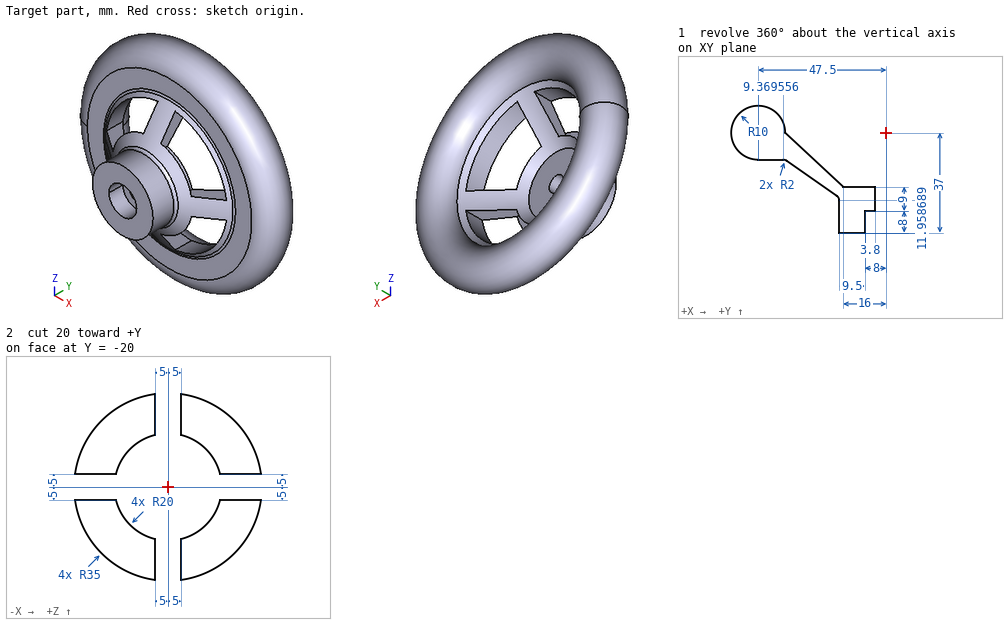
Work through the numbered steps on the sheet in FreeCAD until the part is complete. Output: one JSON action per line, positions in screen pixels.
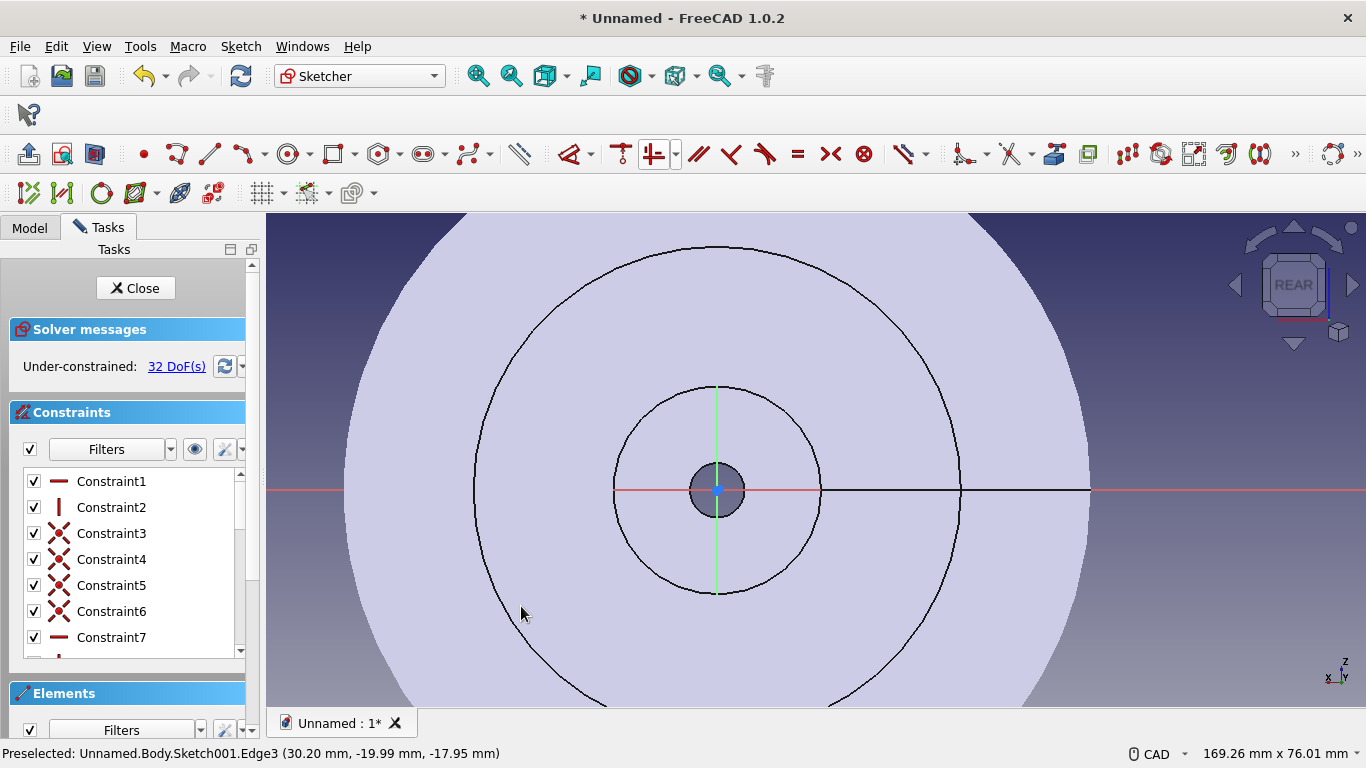
{"action": "left_click", "coordinate": [608, 562]}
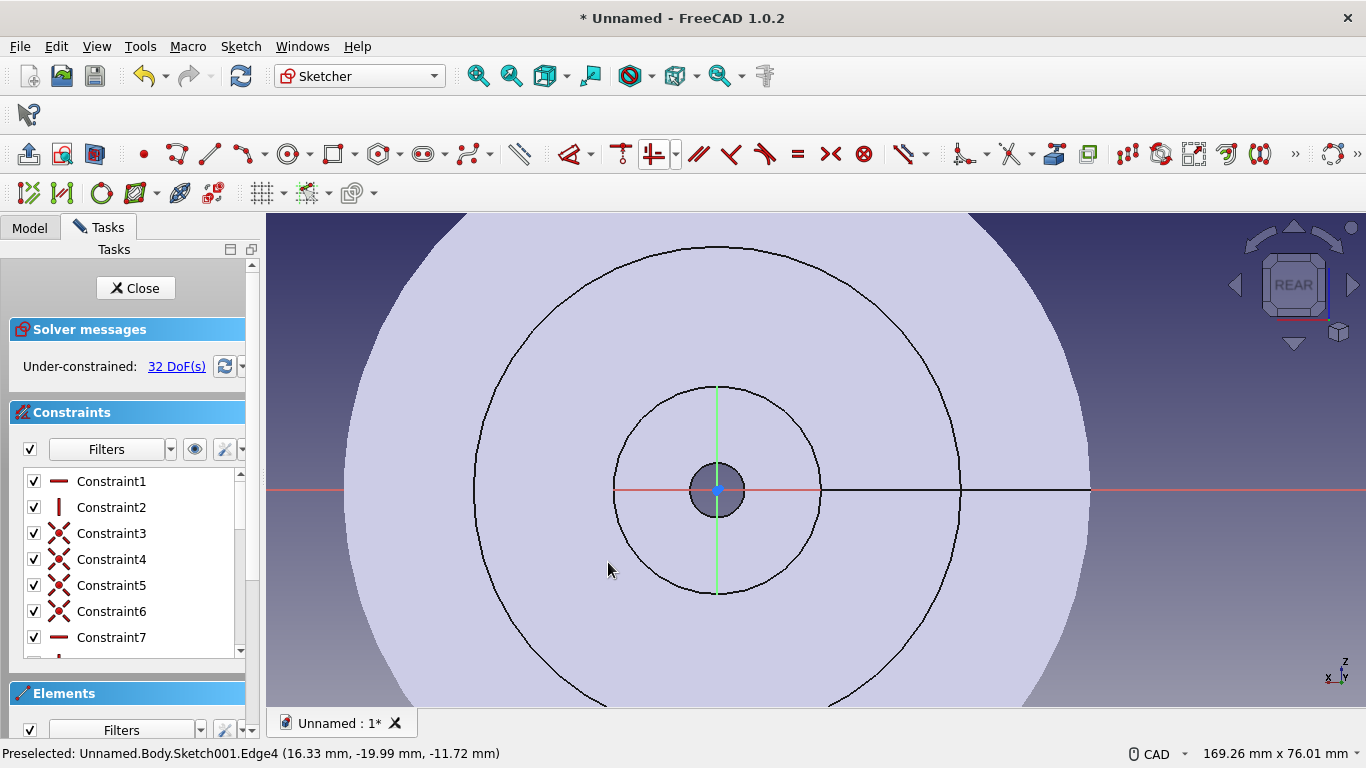
{"action": "key", "text": "c"}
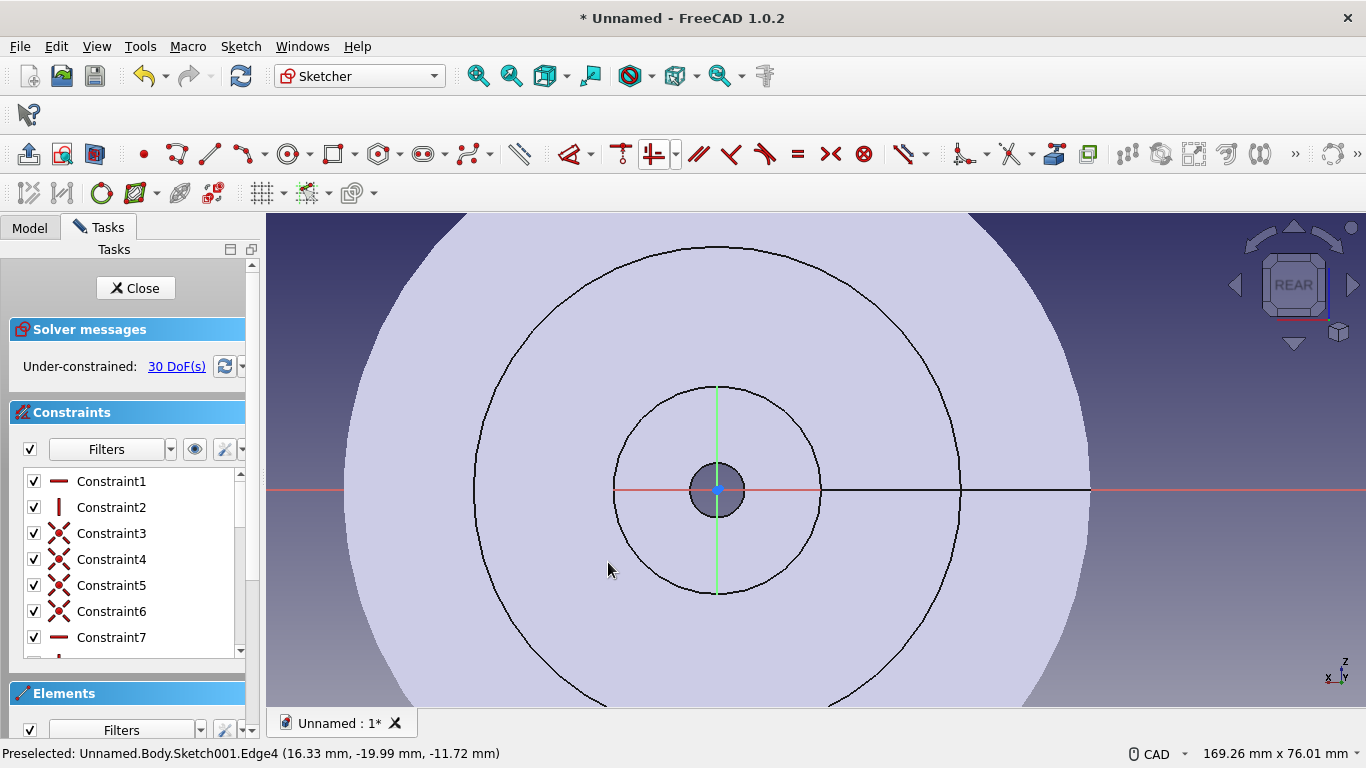
{"action": "left_click", "coordinate": [521, 606]}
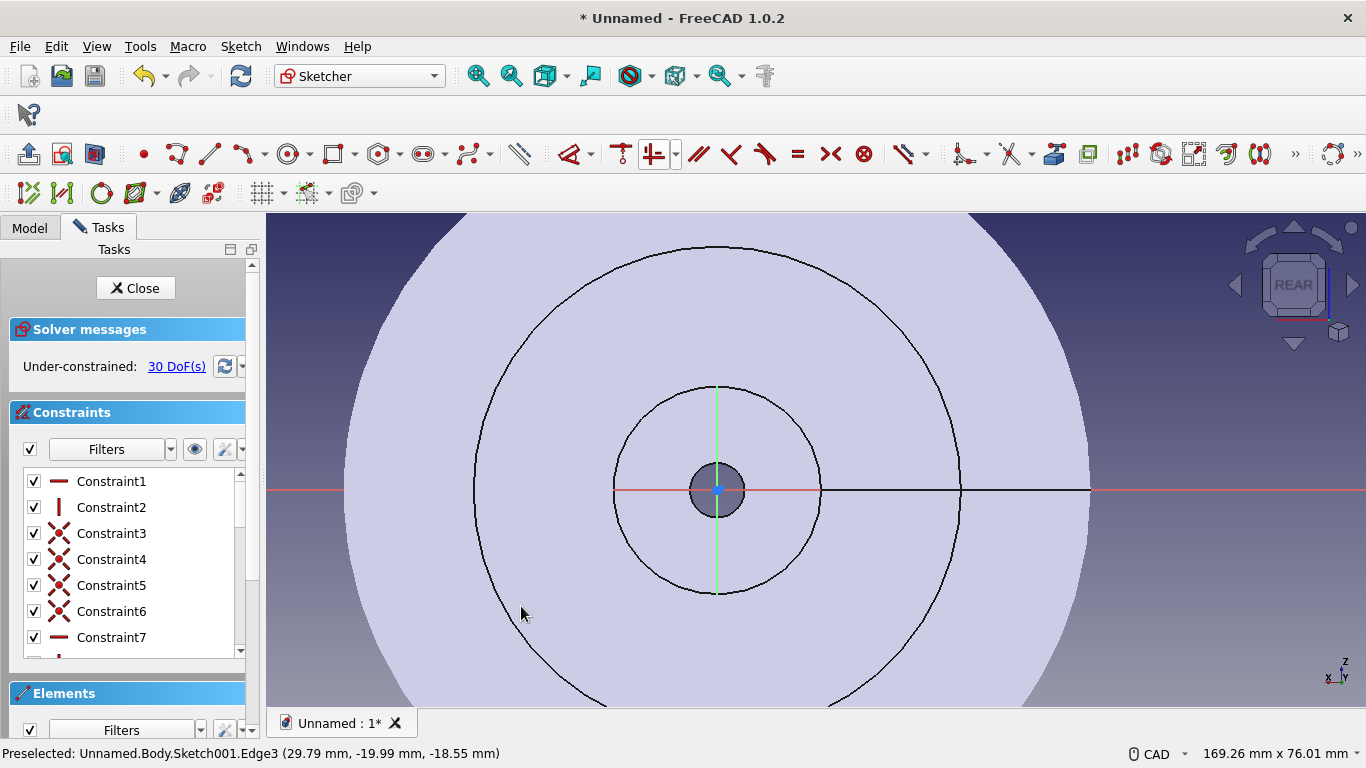
{"action": "left_click", "coordinate": [647, 382]}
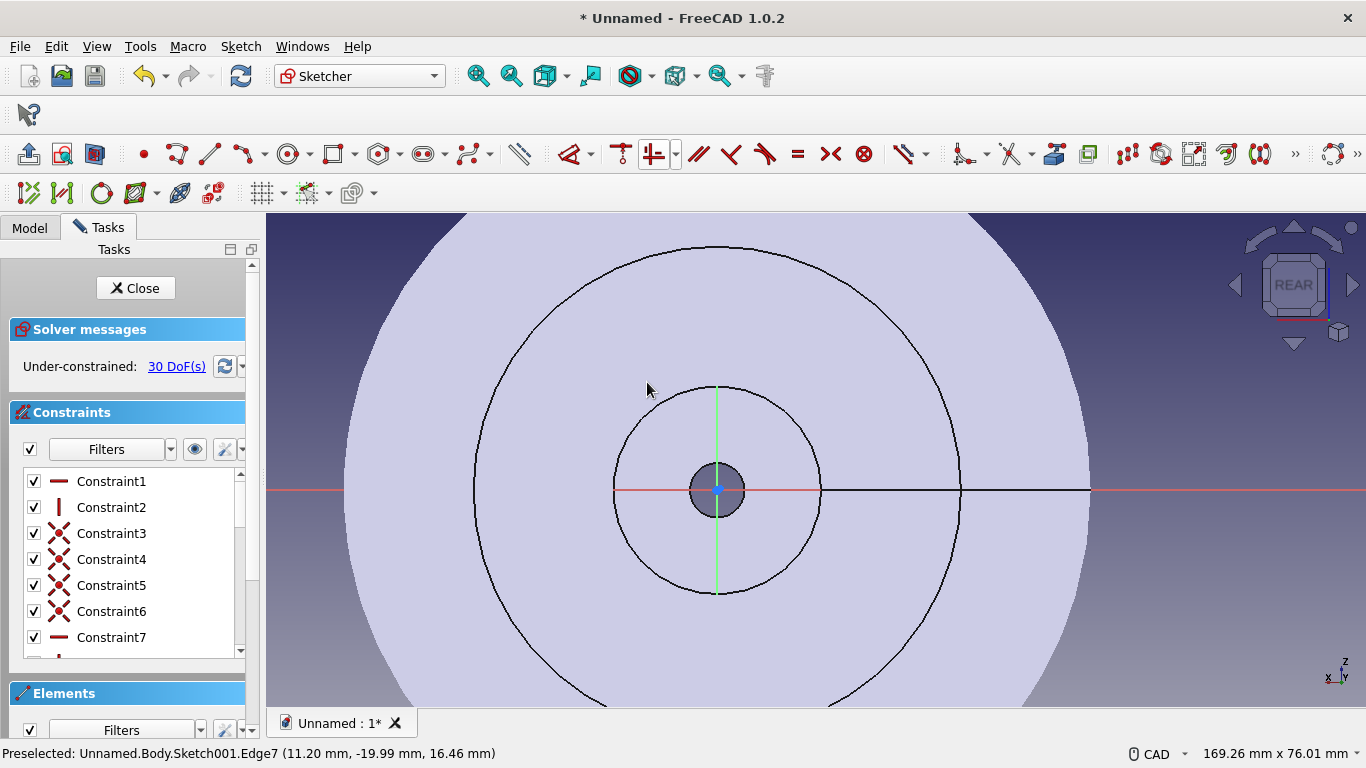
{"action": "key", "text": "c"}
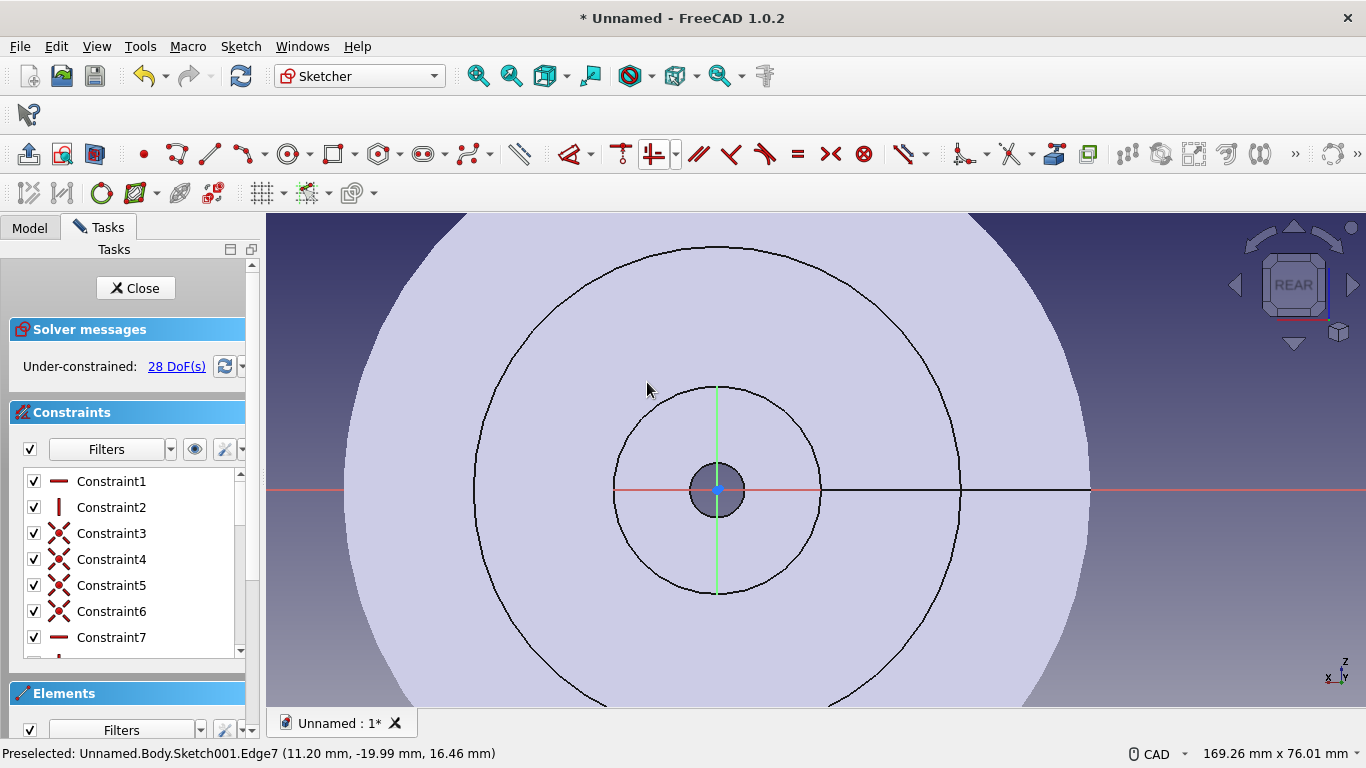
{"action": "left_click", "coordinate": [521, 606]}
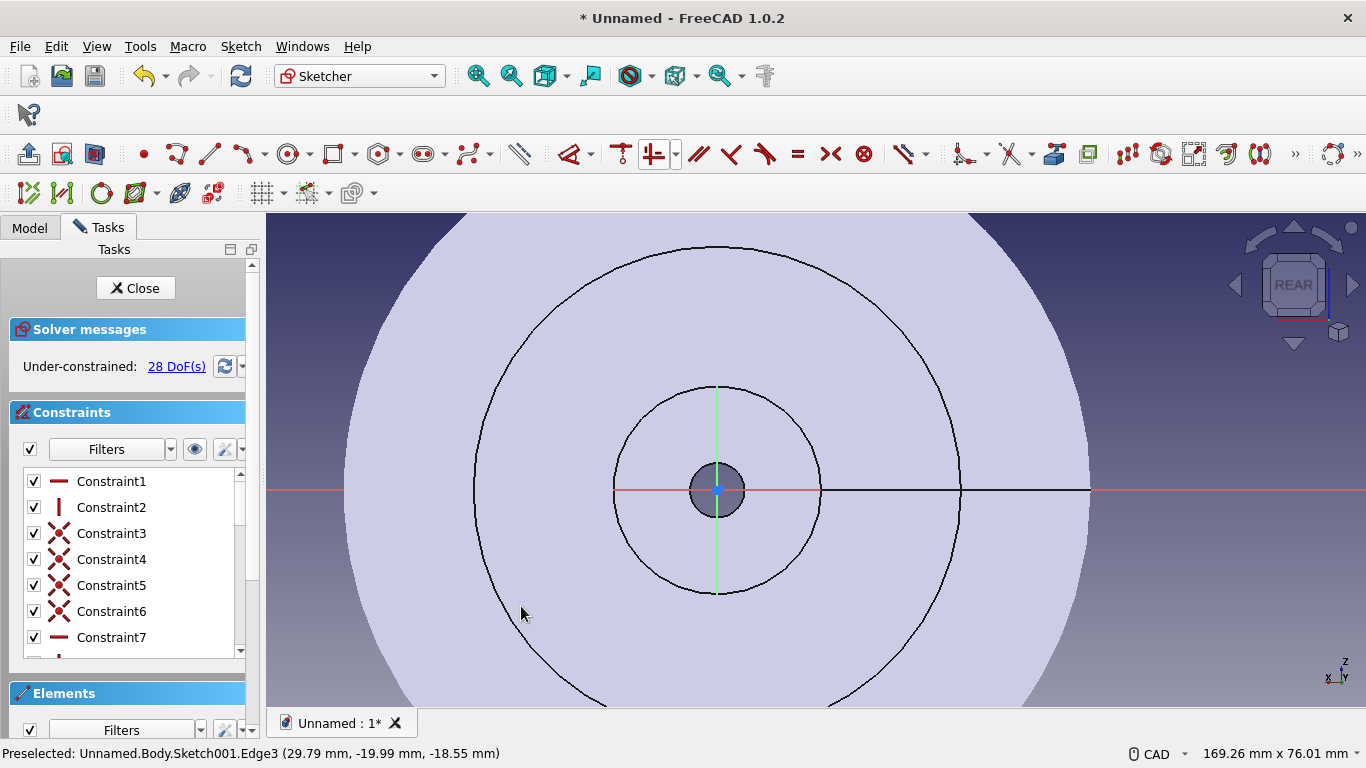
{"action": "left_click", "coordinate": [602, 295]}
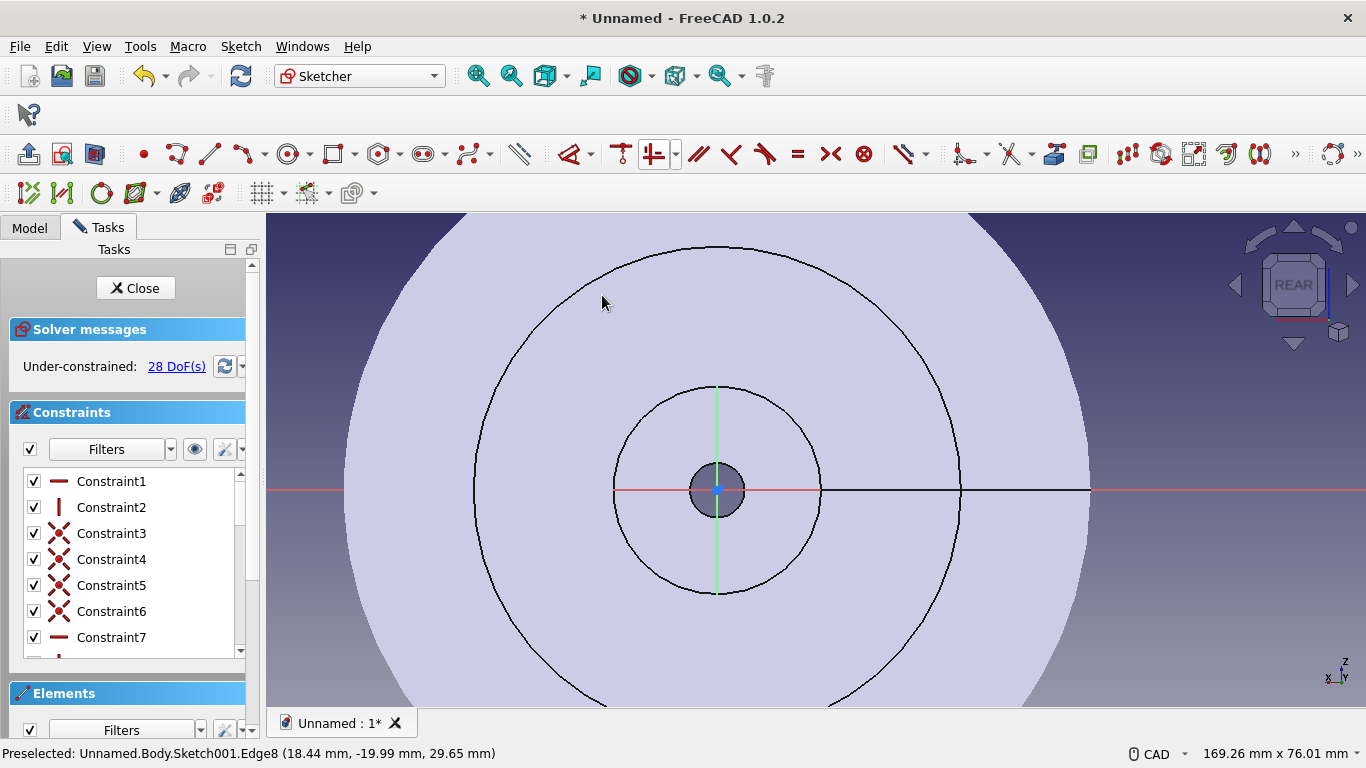
{"action": "key", "text": "c"}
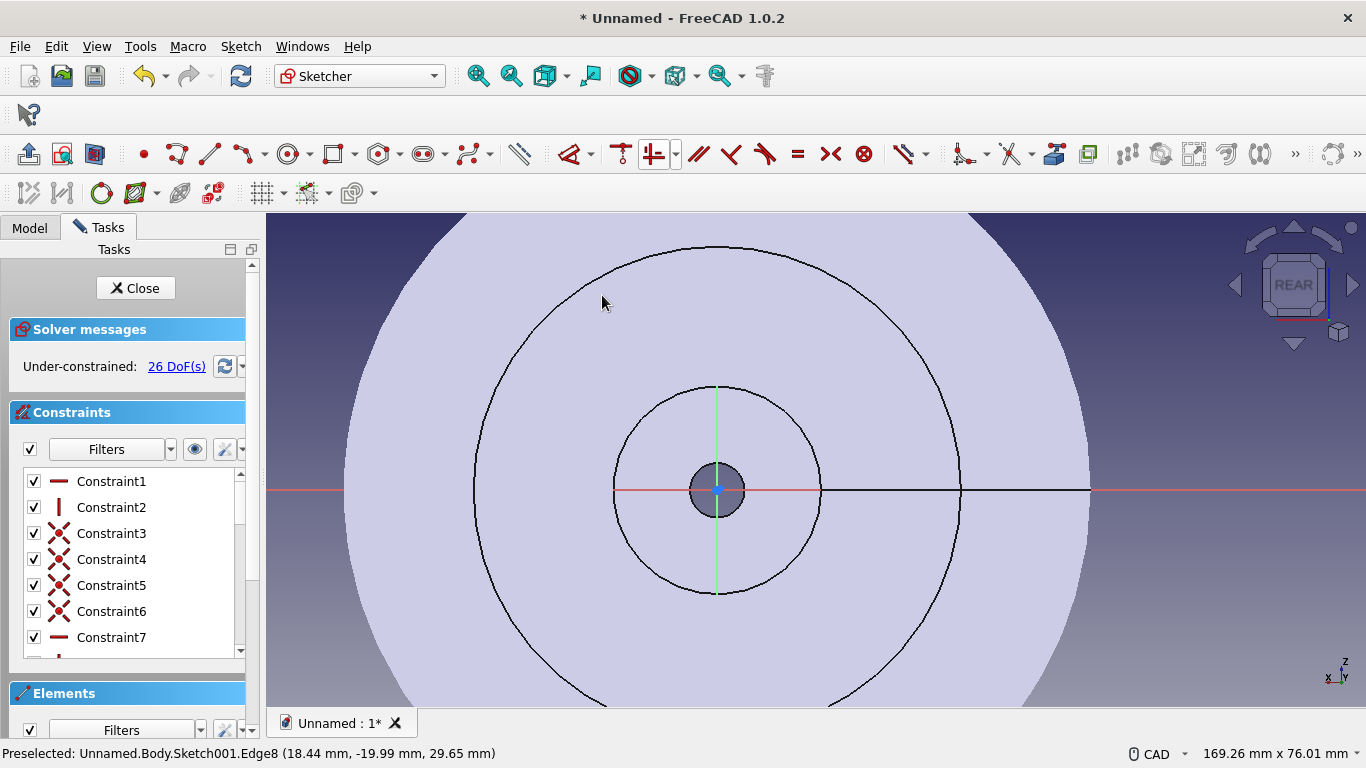
{"action": "left_click", "coordinate": [520, 606]}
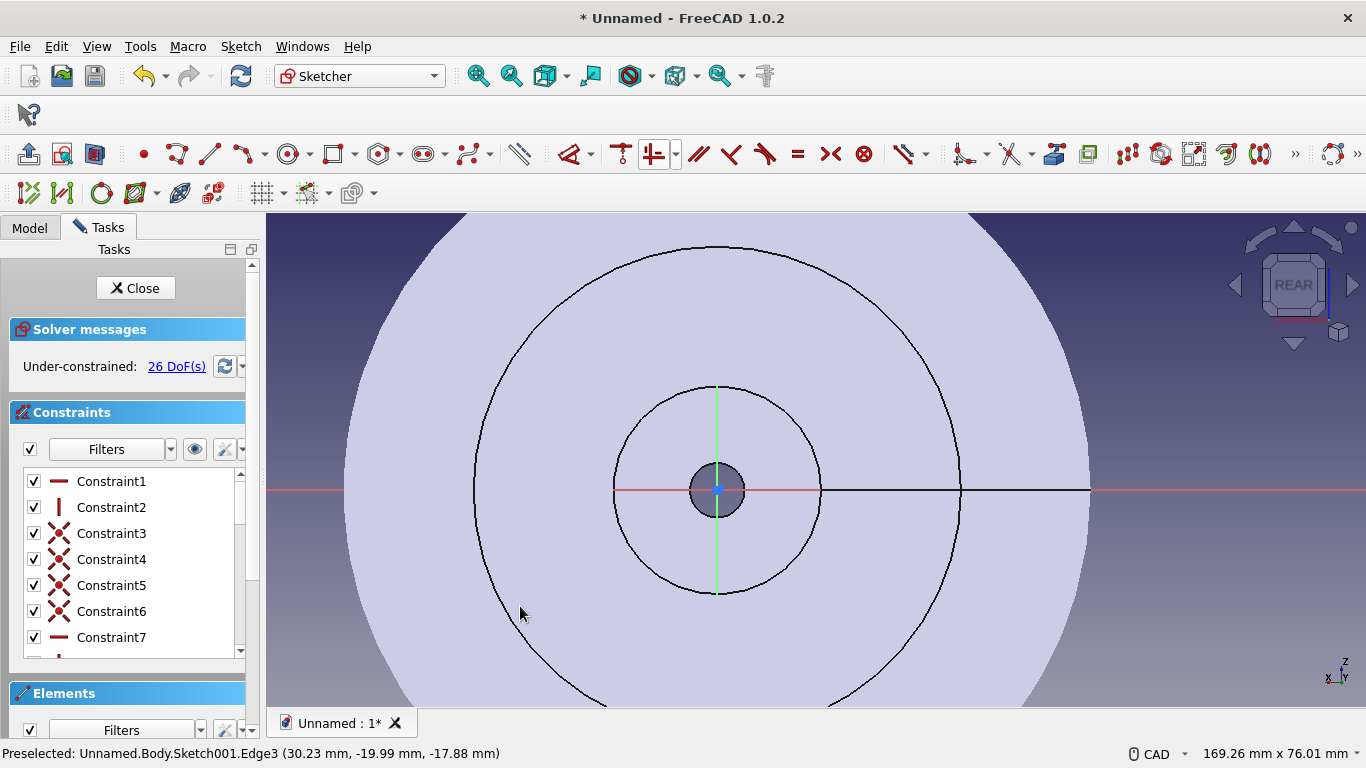
{"action": "left_click", "coordinate": [787, 600]}